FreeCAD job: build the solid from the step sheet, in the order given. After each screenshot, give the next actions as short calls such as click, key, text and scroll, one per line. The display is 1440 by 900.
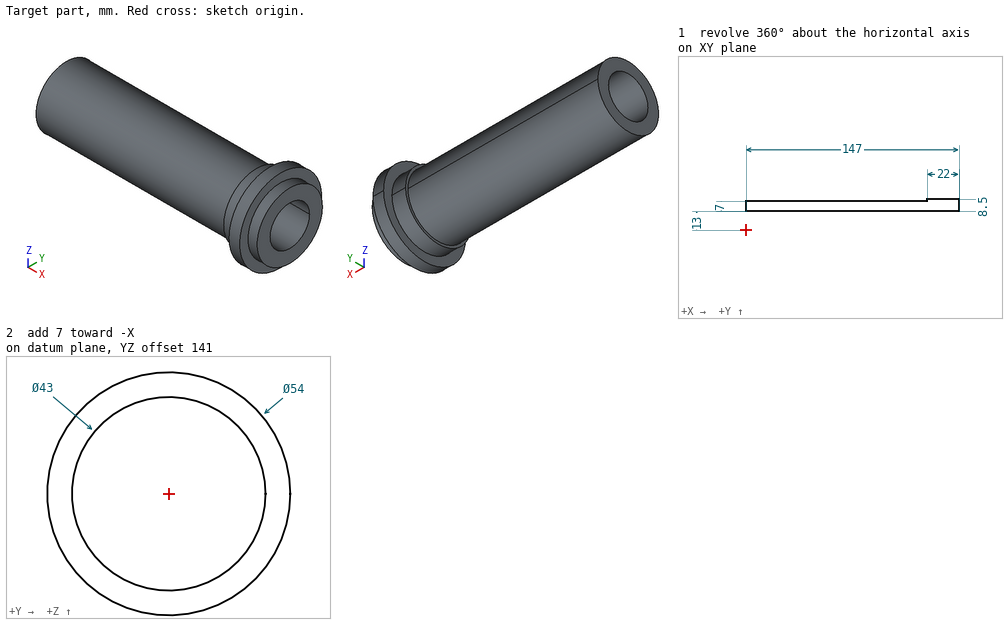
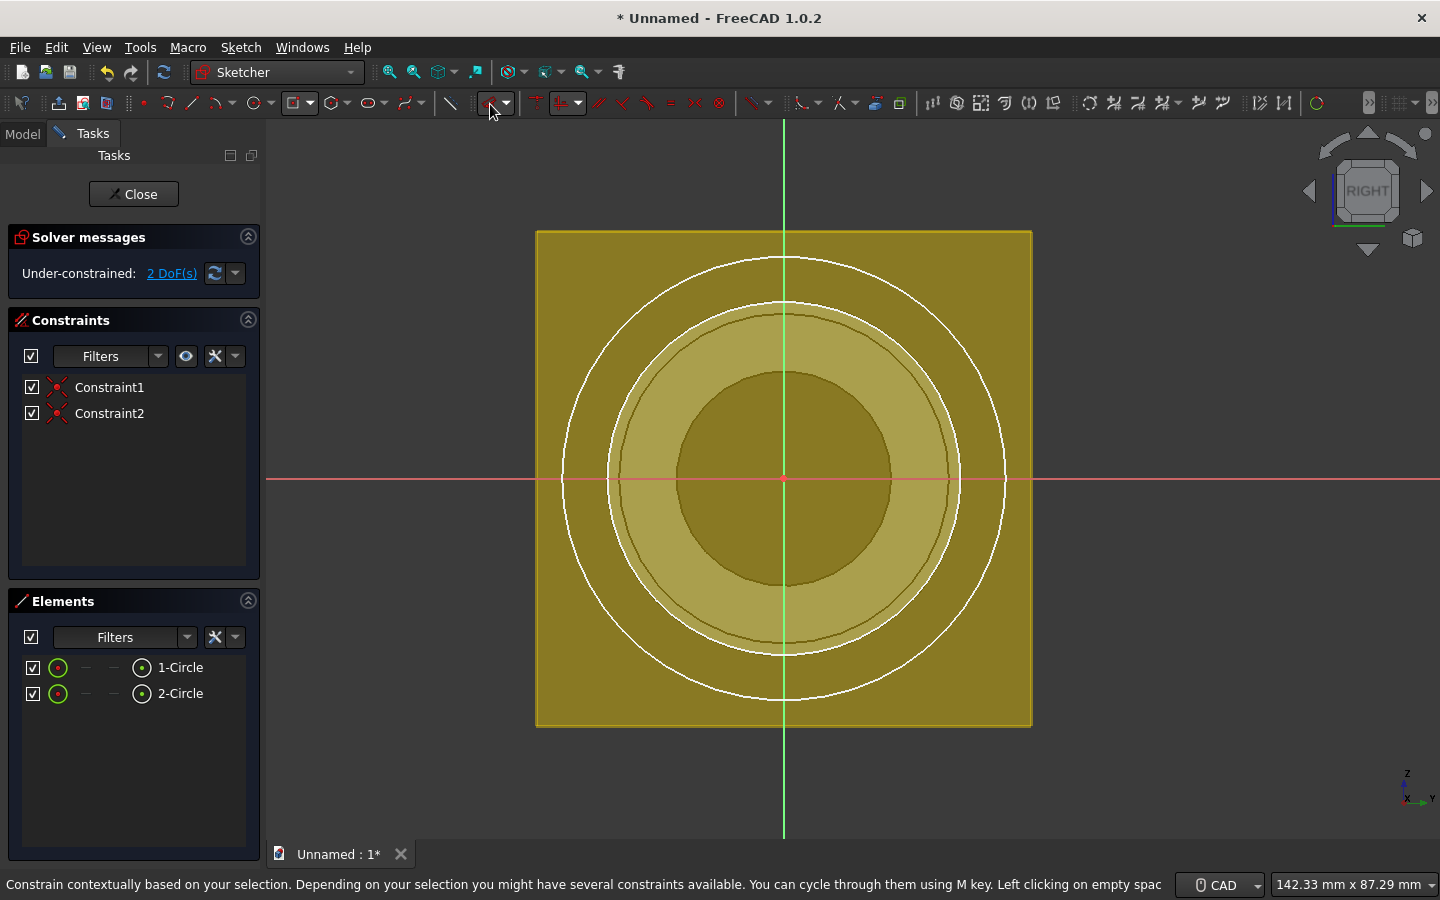
click(940, 321)
click(963, 298)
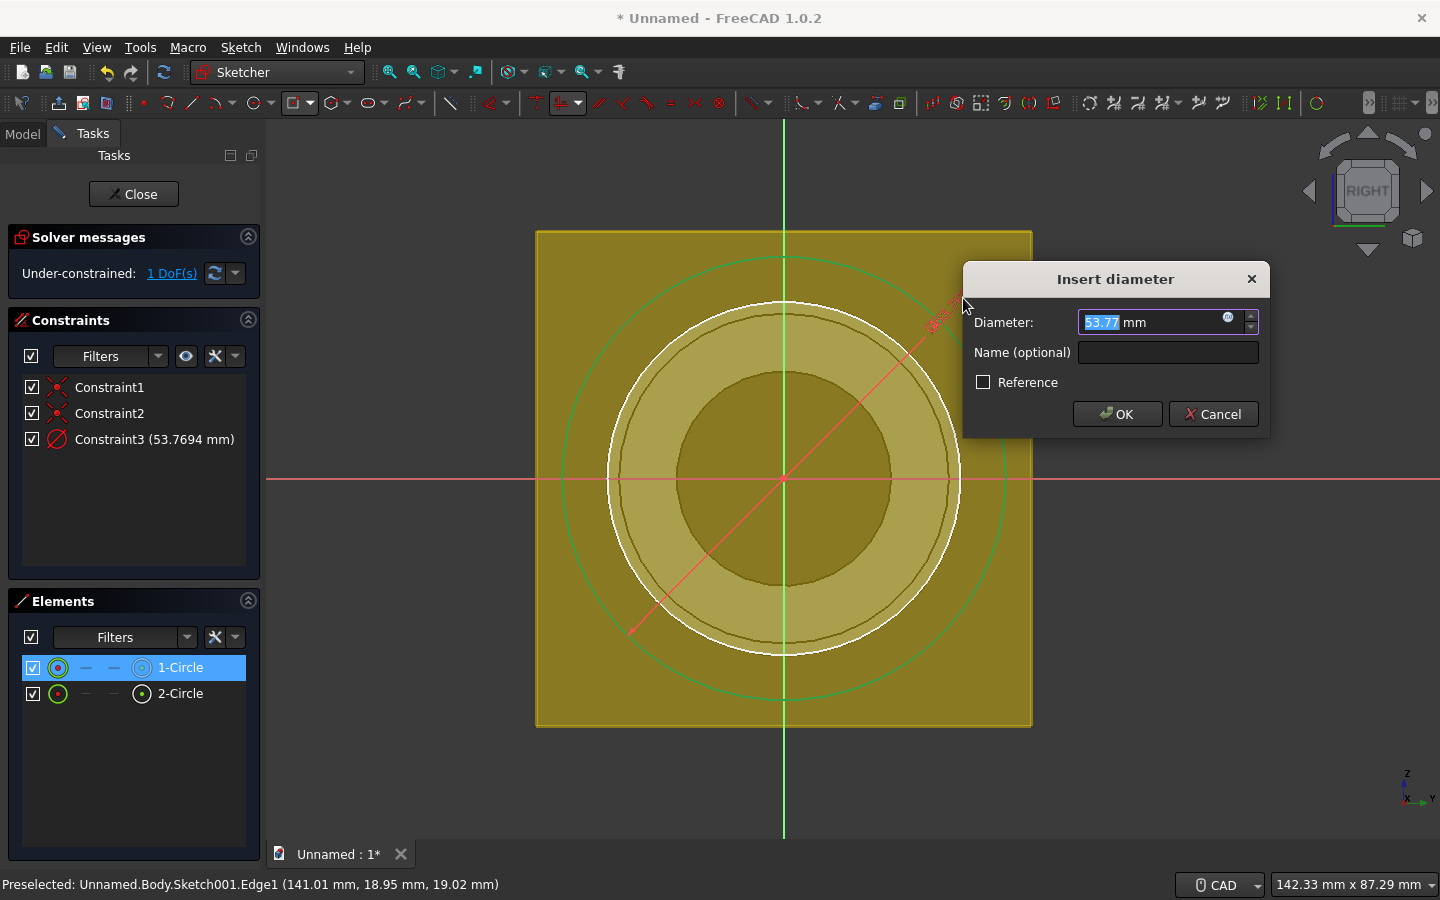
text(54)
key(Return)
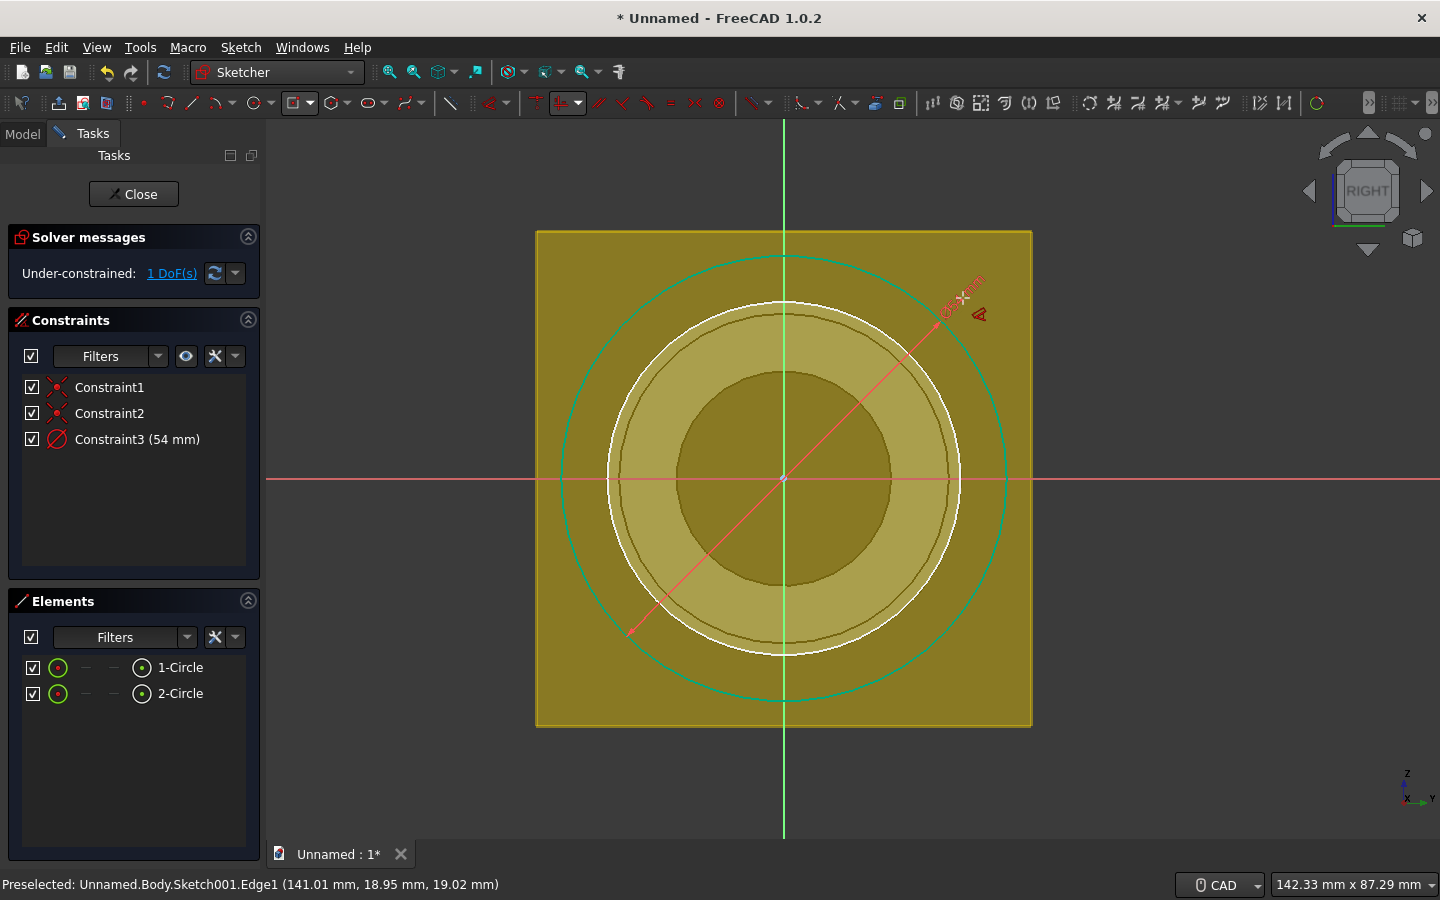
click(908, 353)
click(930, 330)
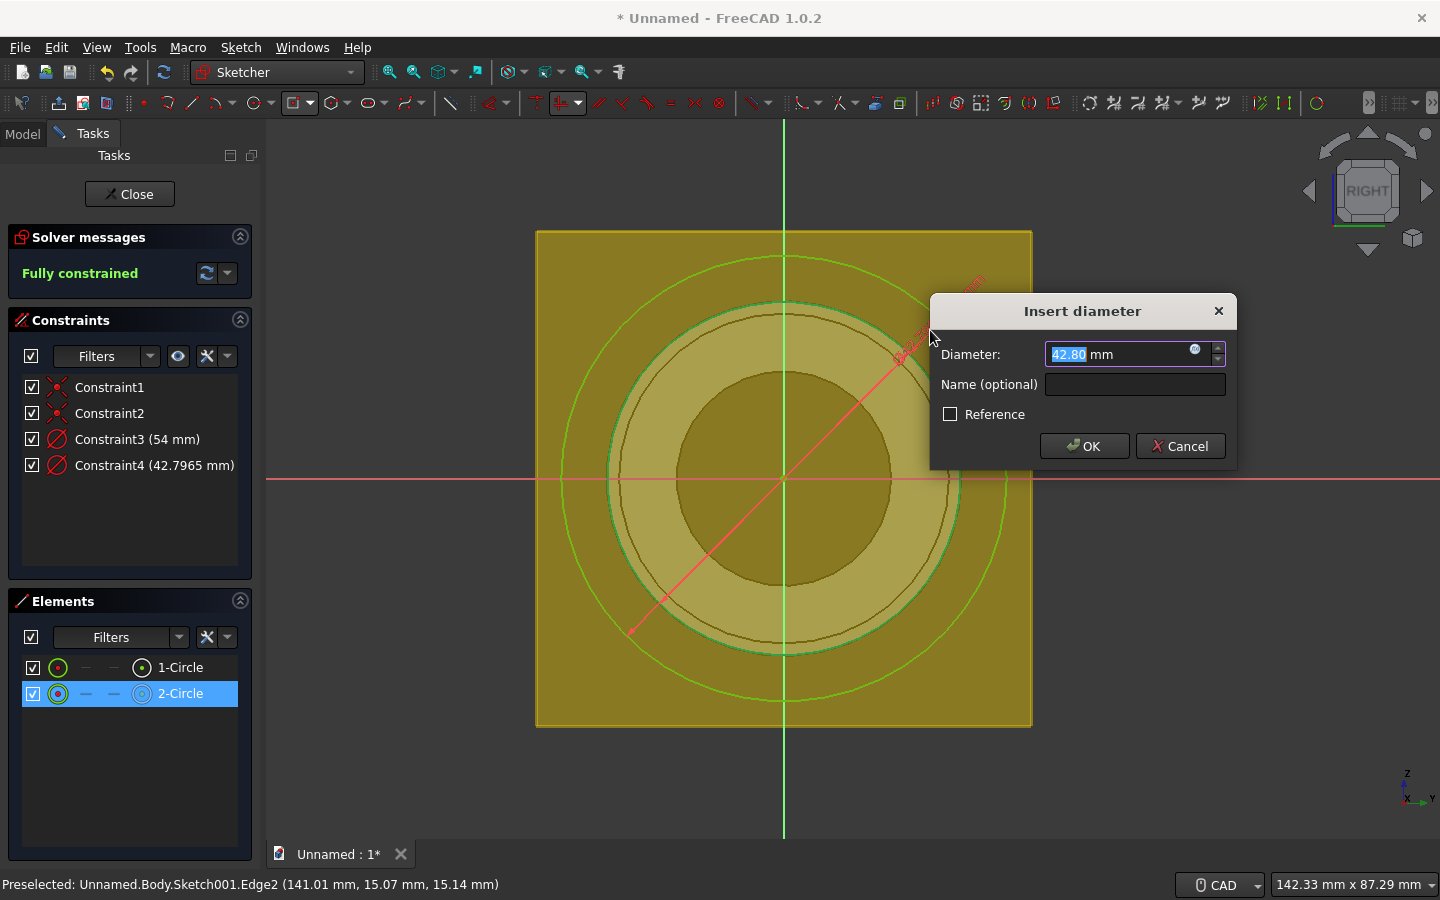
text(43)
key(Return)
key(Escape)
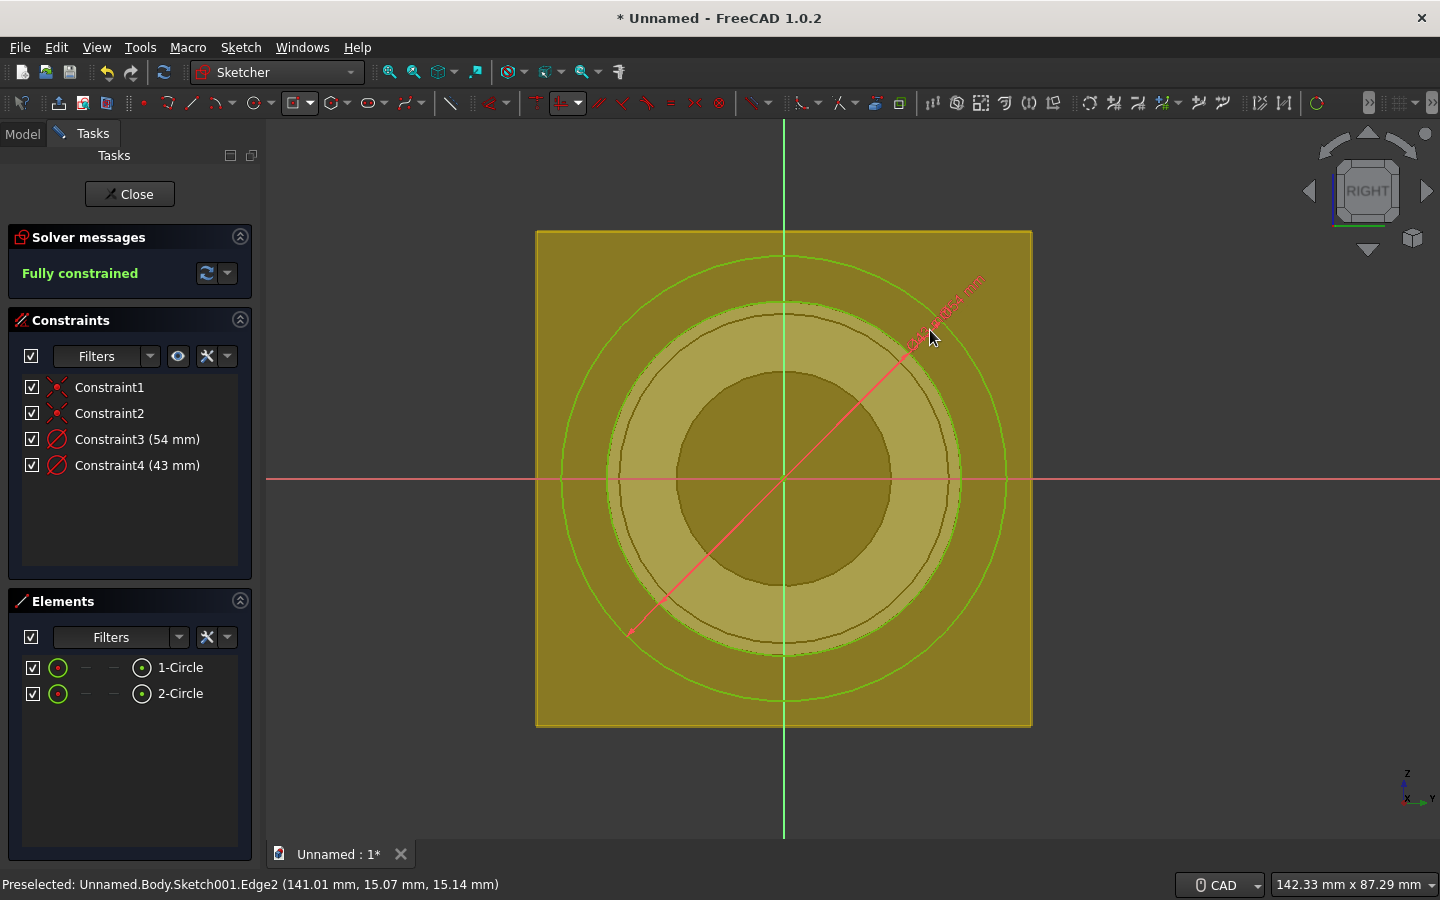
click(130, 194)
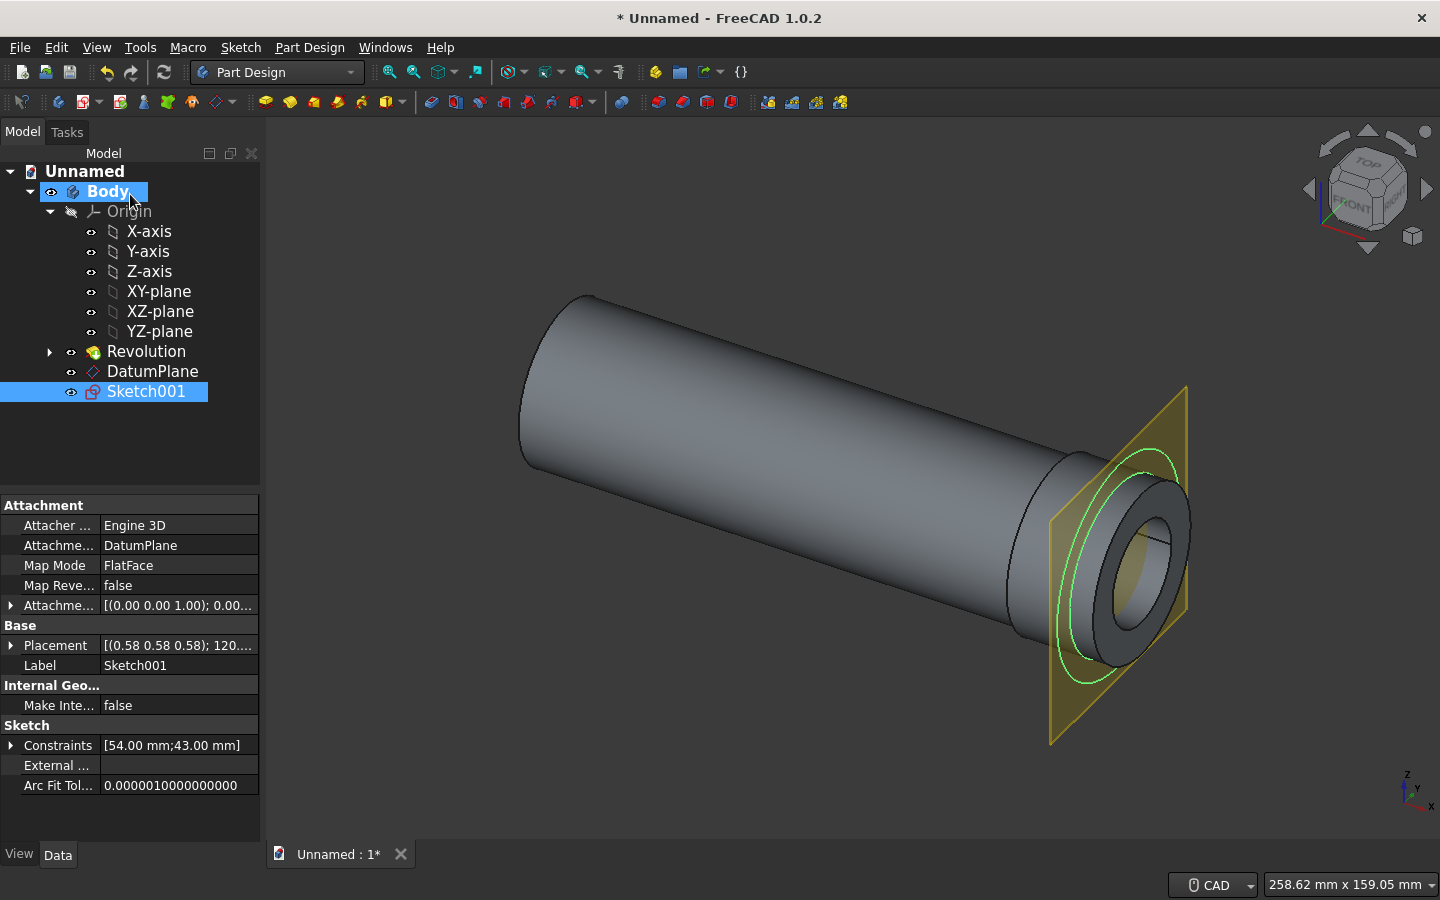
click(266, 102)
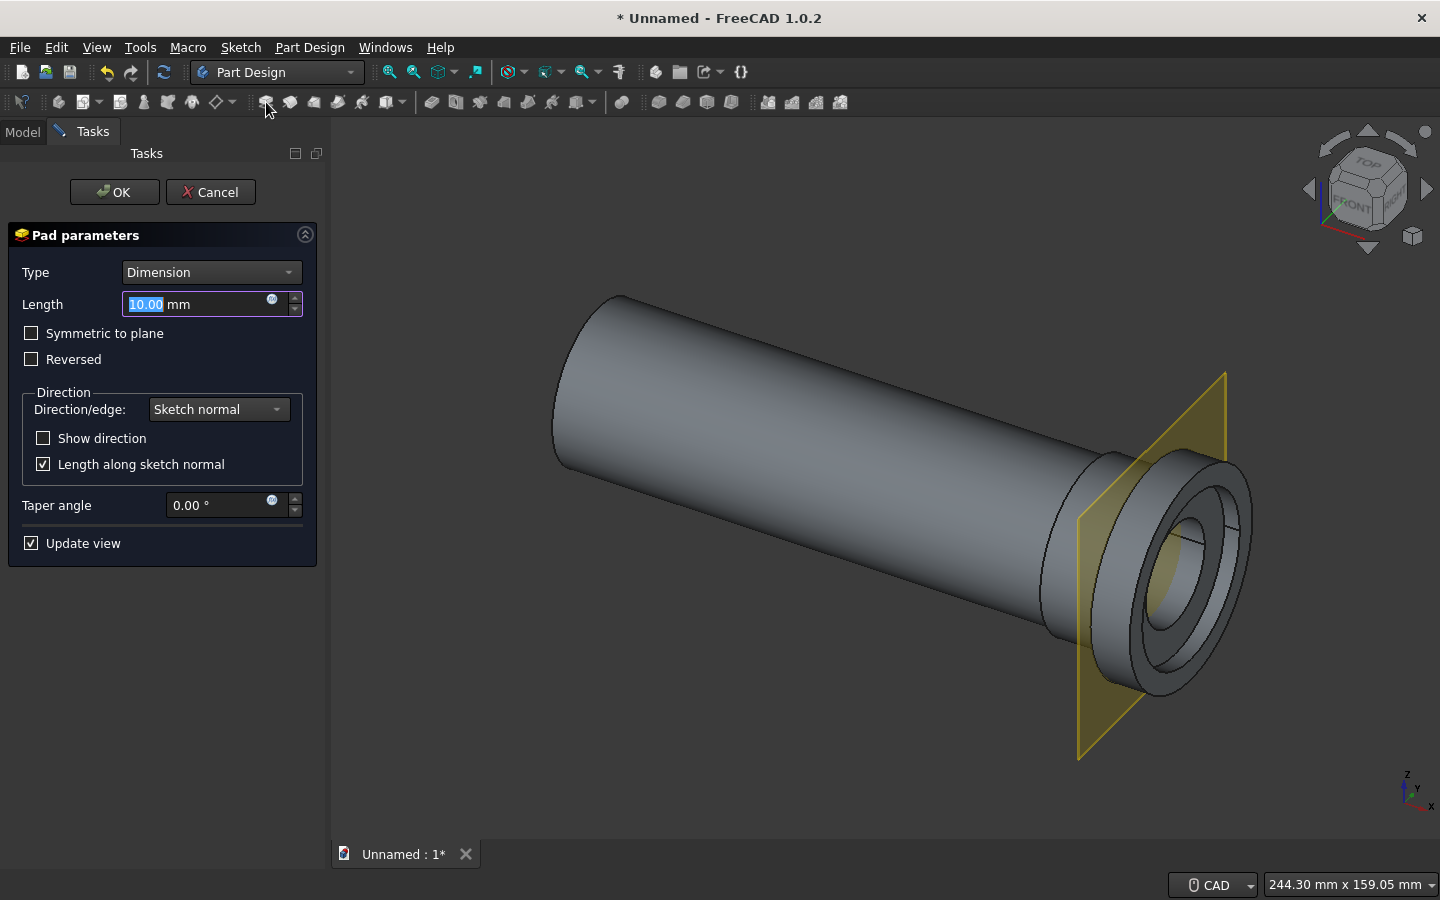
text(7)
key(Tab)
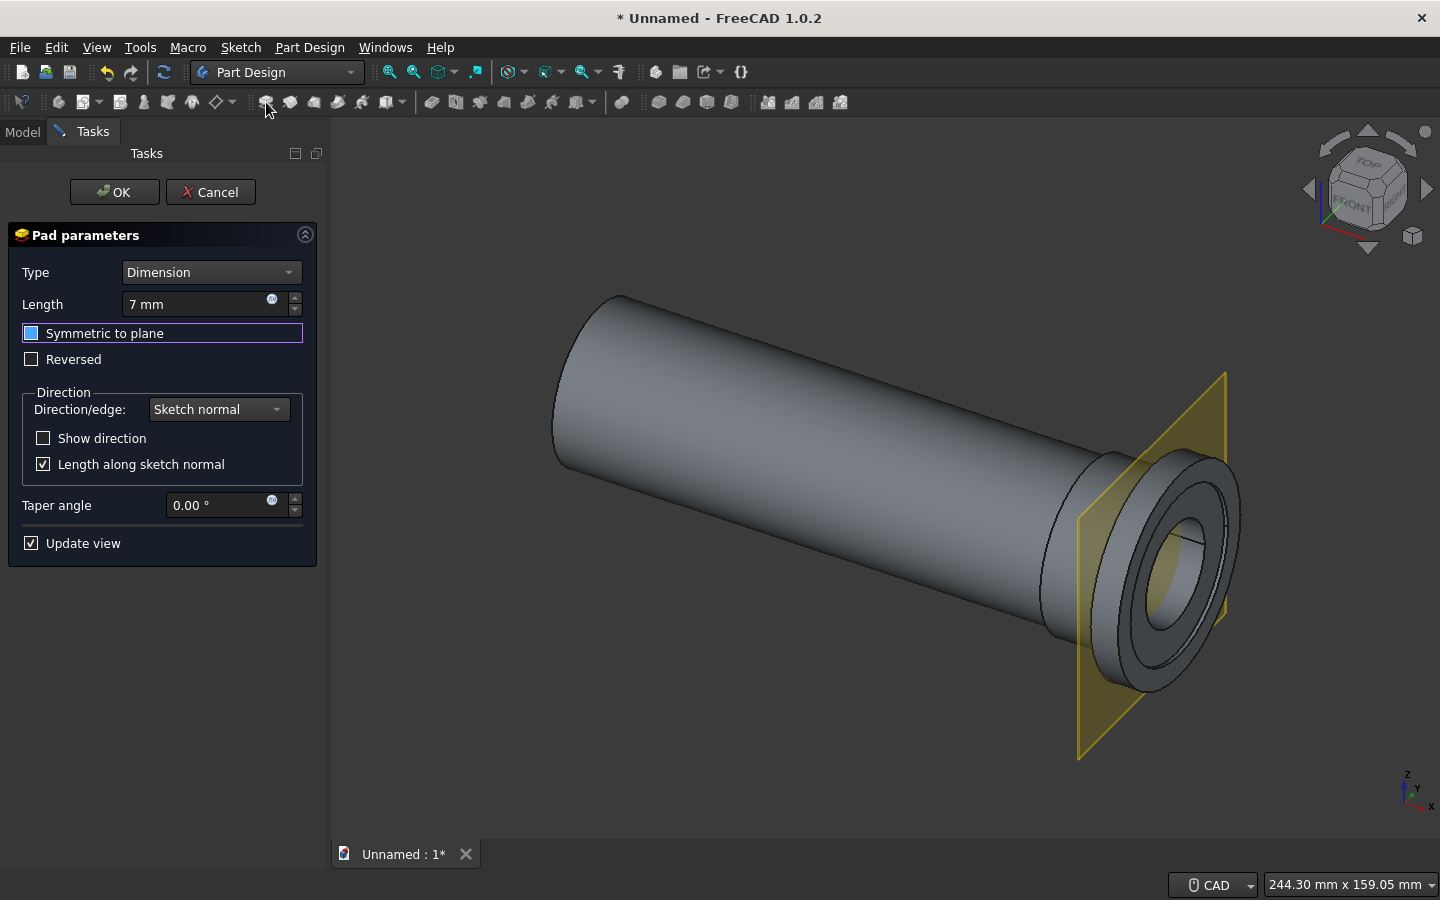
click(30, 359)